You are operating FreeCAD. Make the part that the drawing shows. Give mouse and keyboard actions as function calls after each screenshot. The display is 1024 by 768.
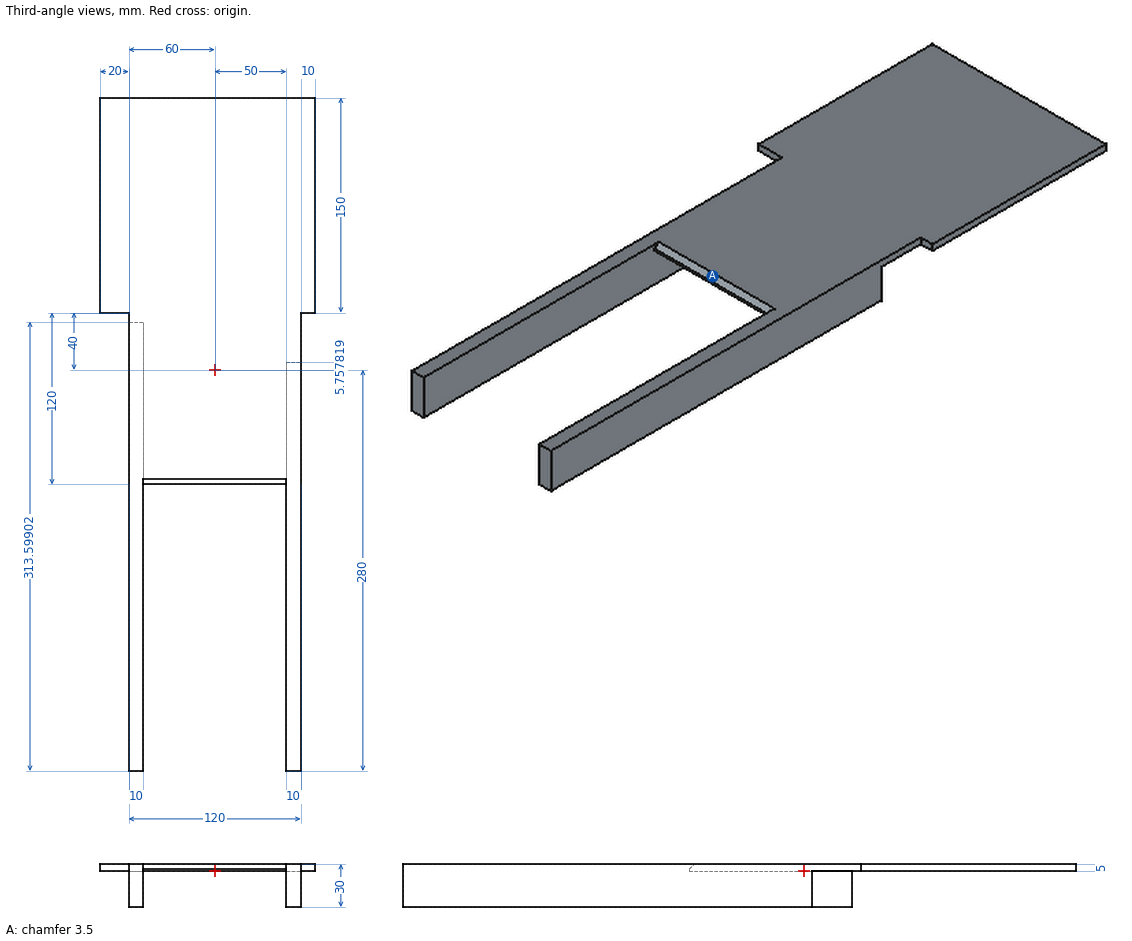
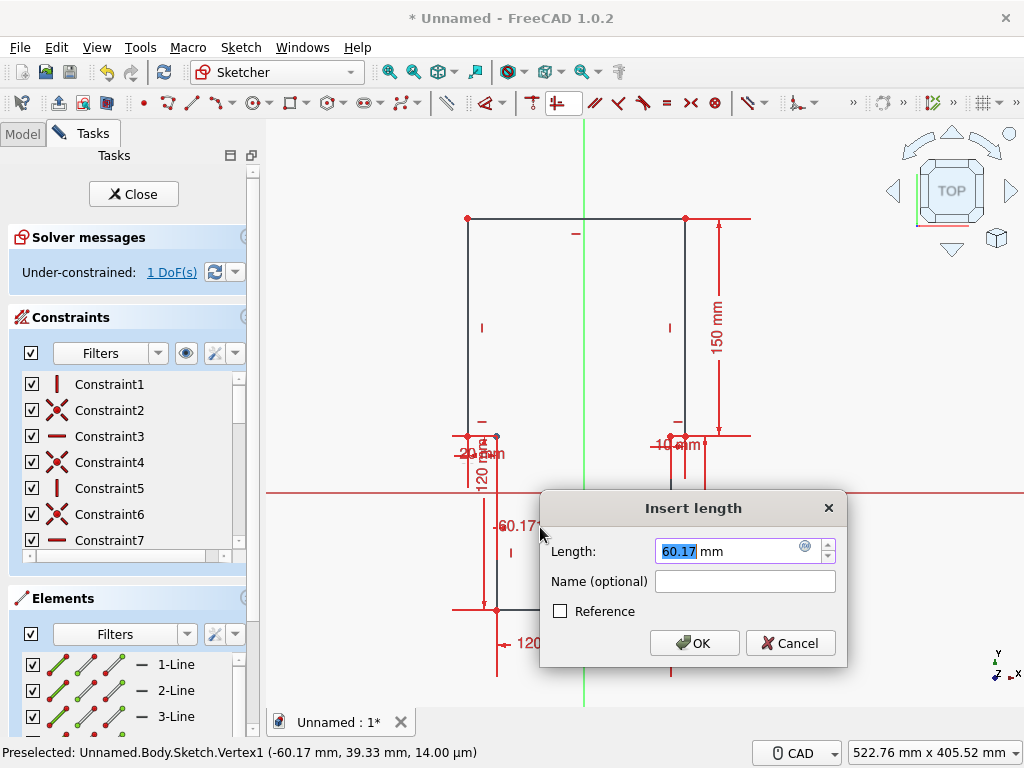
text(60)
key(Return)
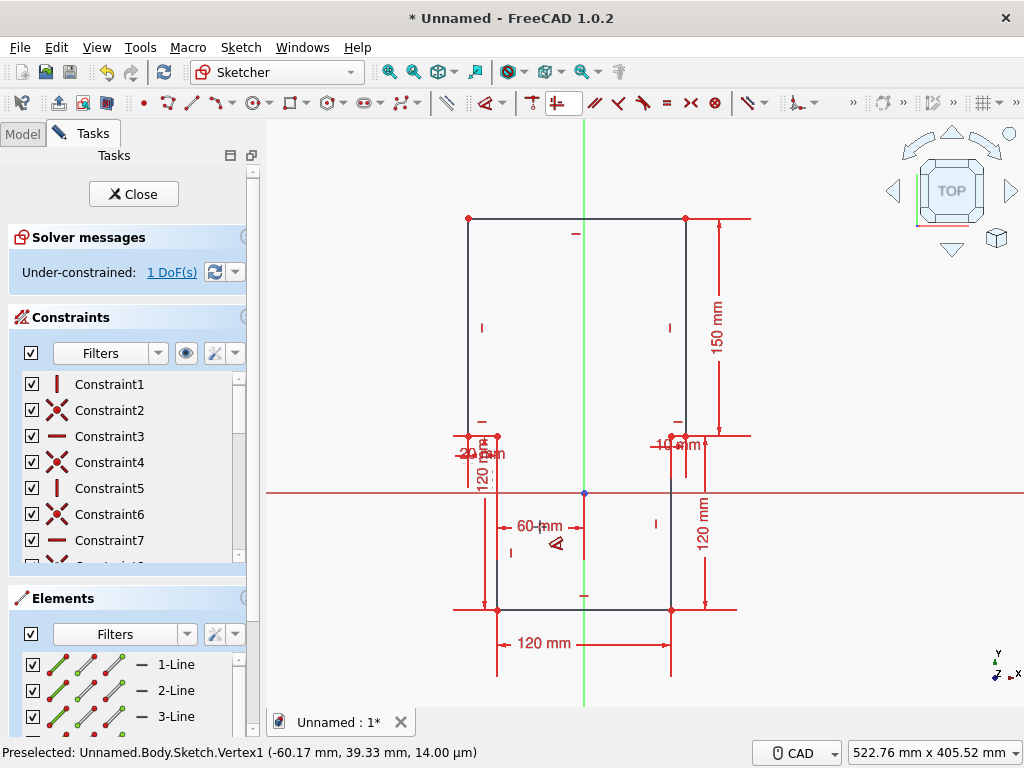
click(497, 436)
click(618, 478)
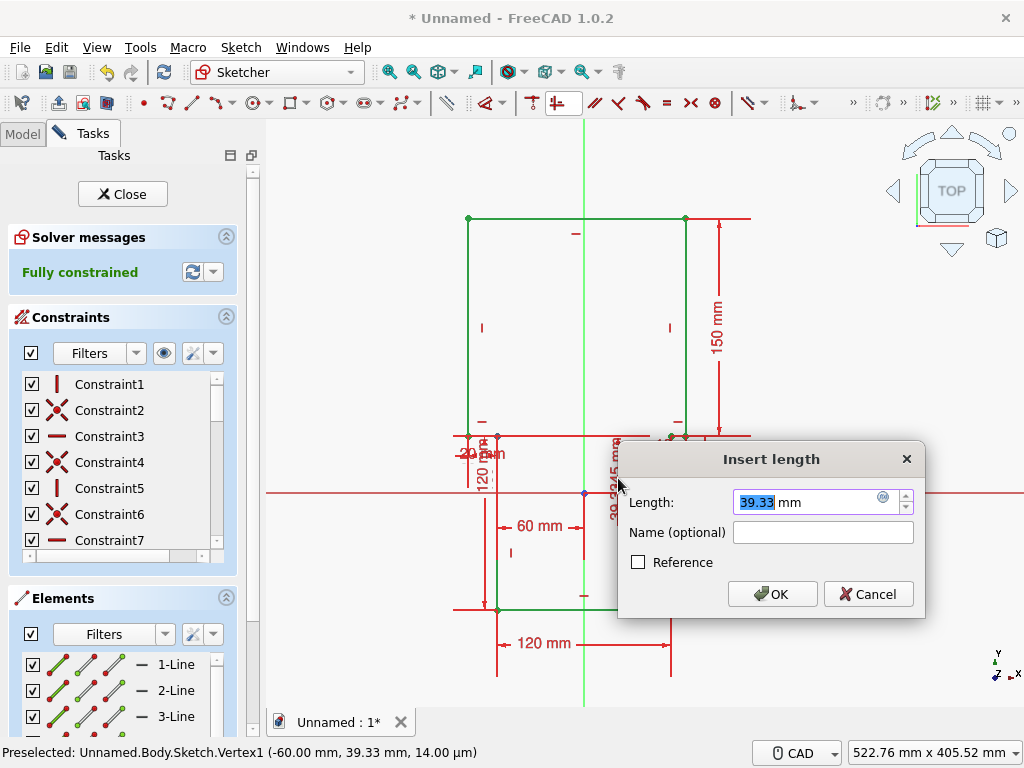
text(40)
key(Return)
key(Escape)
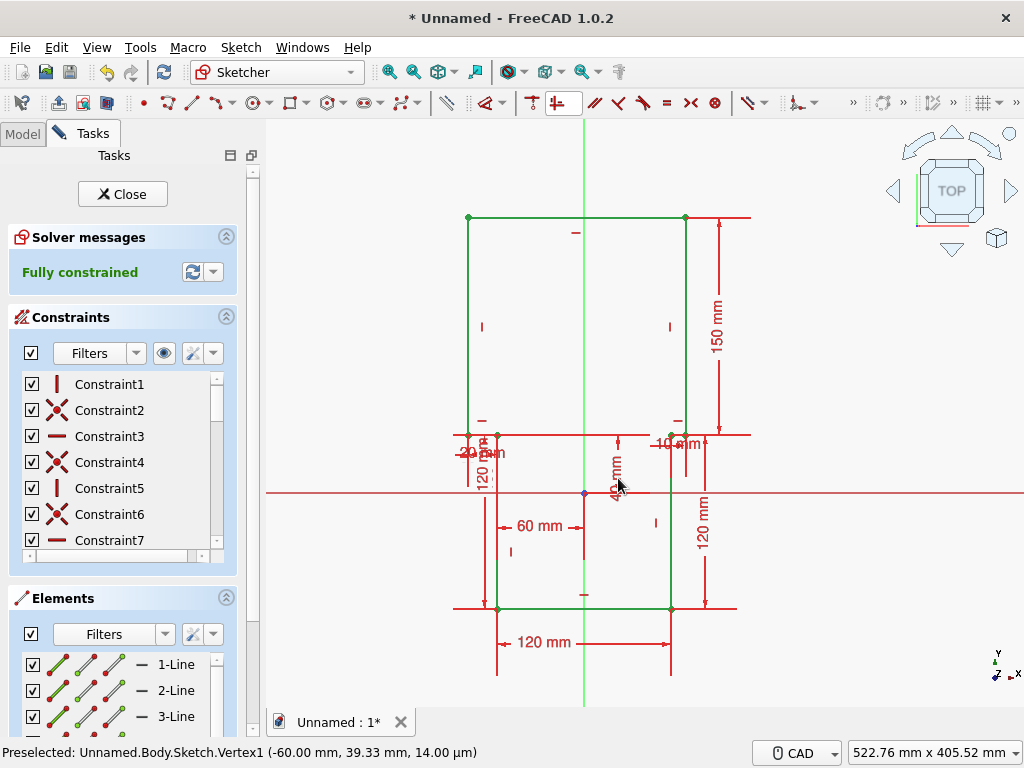
click(123, 194)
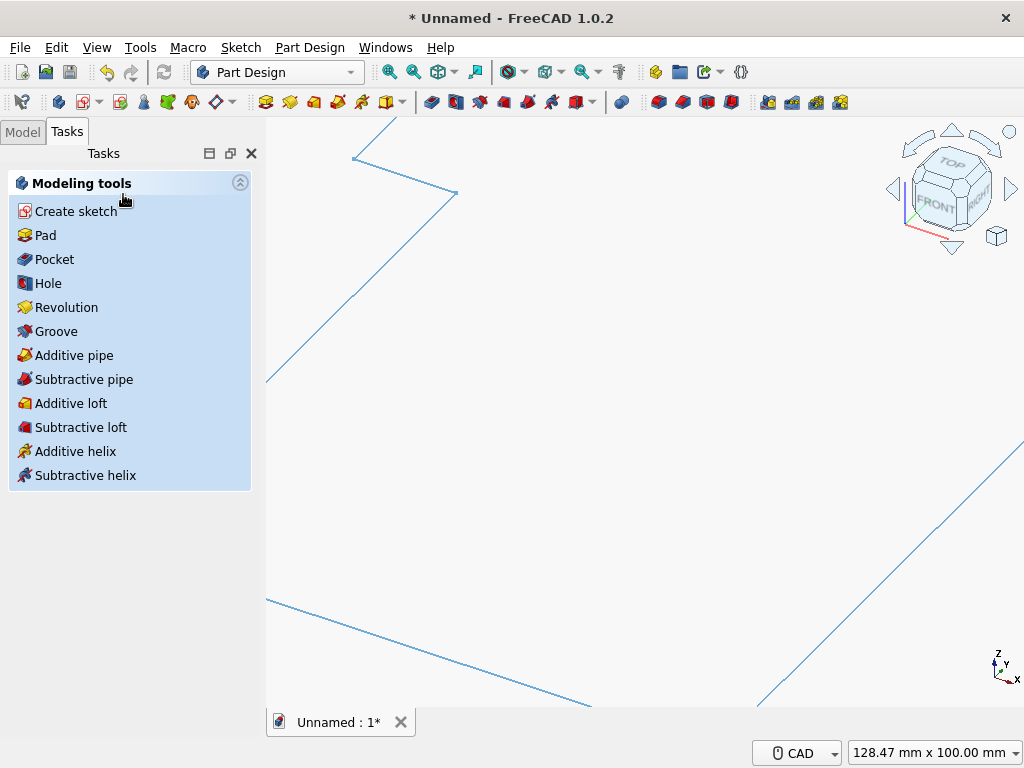
click(266, 102)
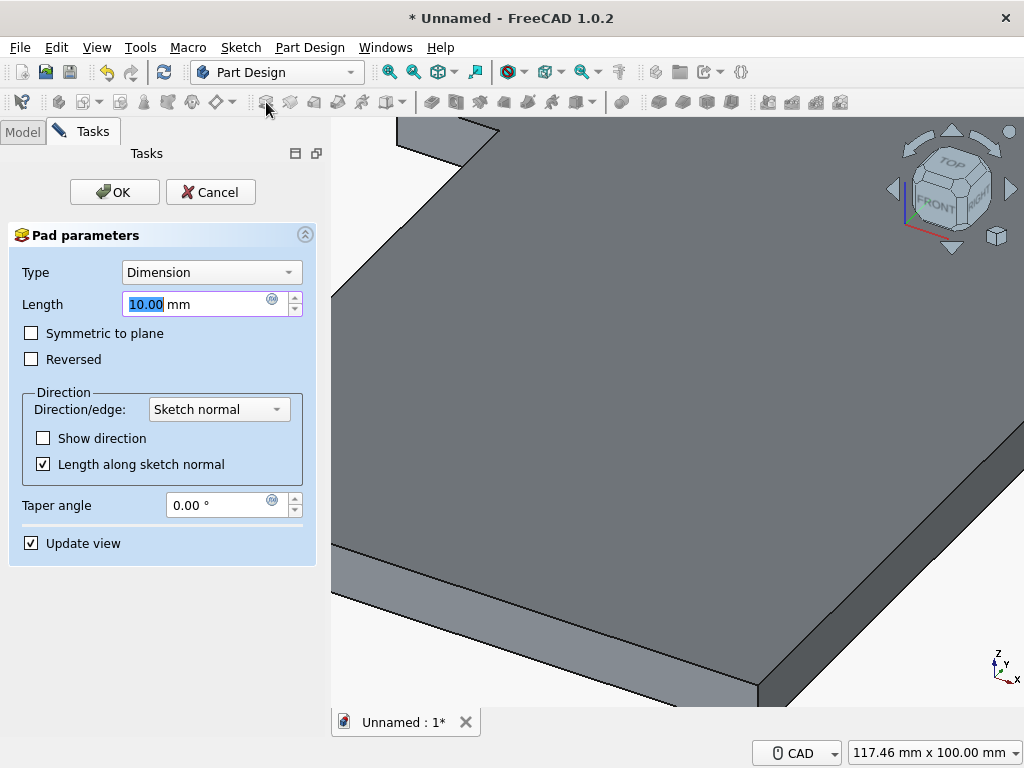
text(5)
key(Tab)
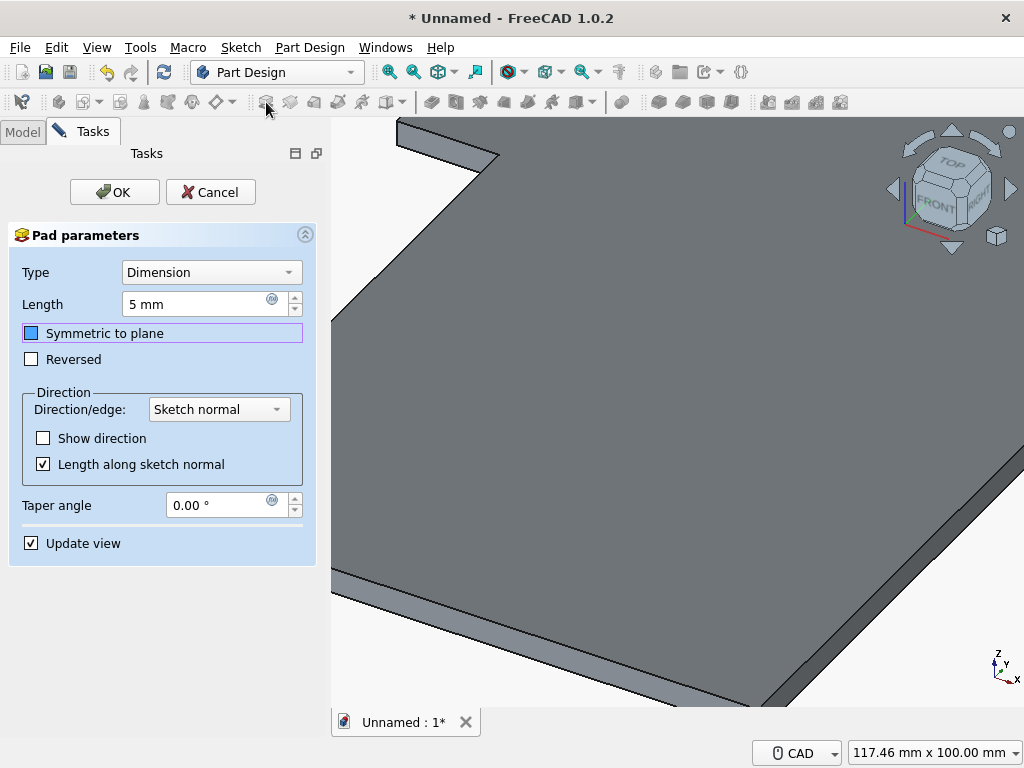
click(115, 192)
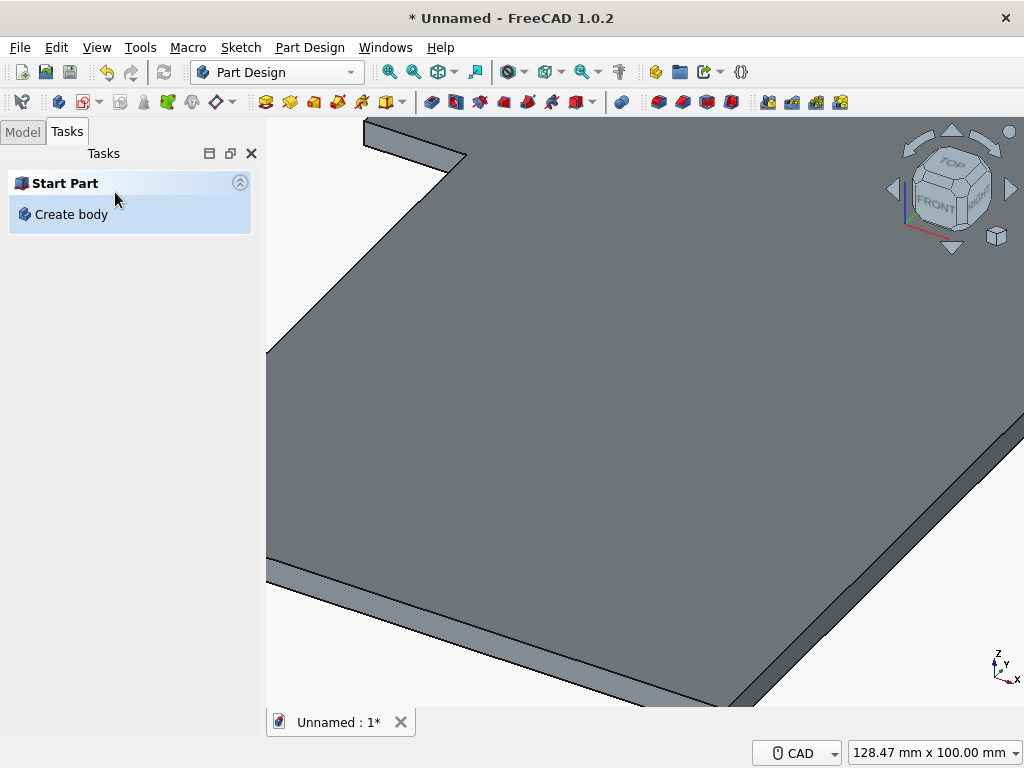
click(390, 72)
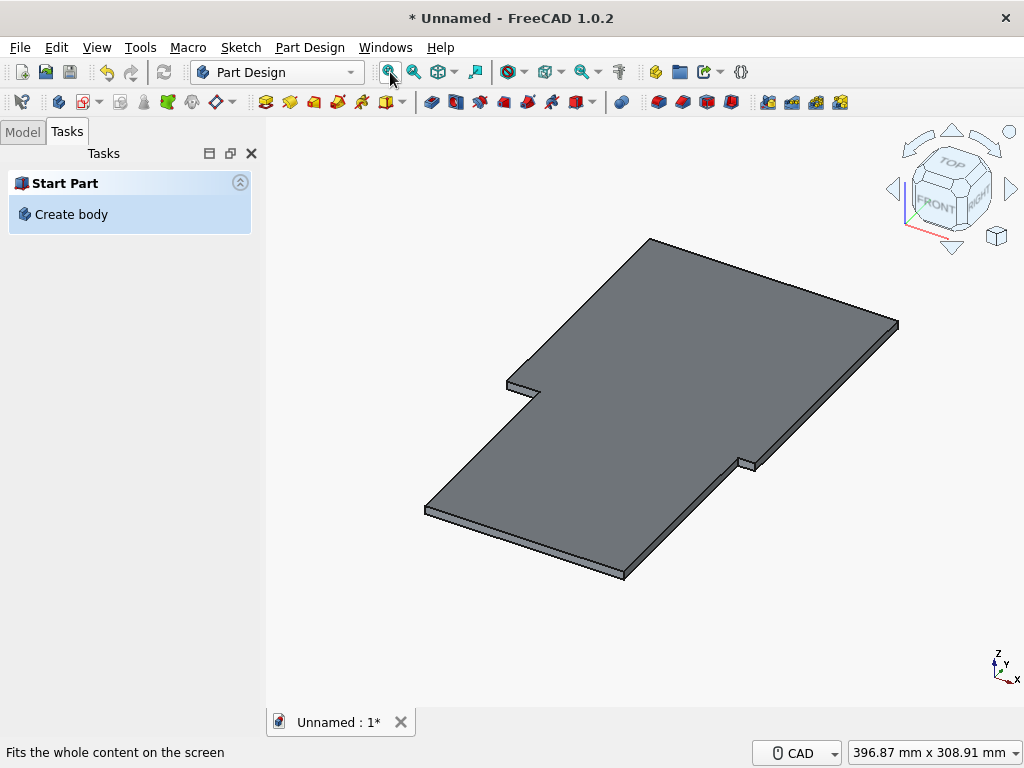
click(682, 370)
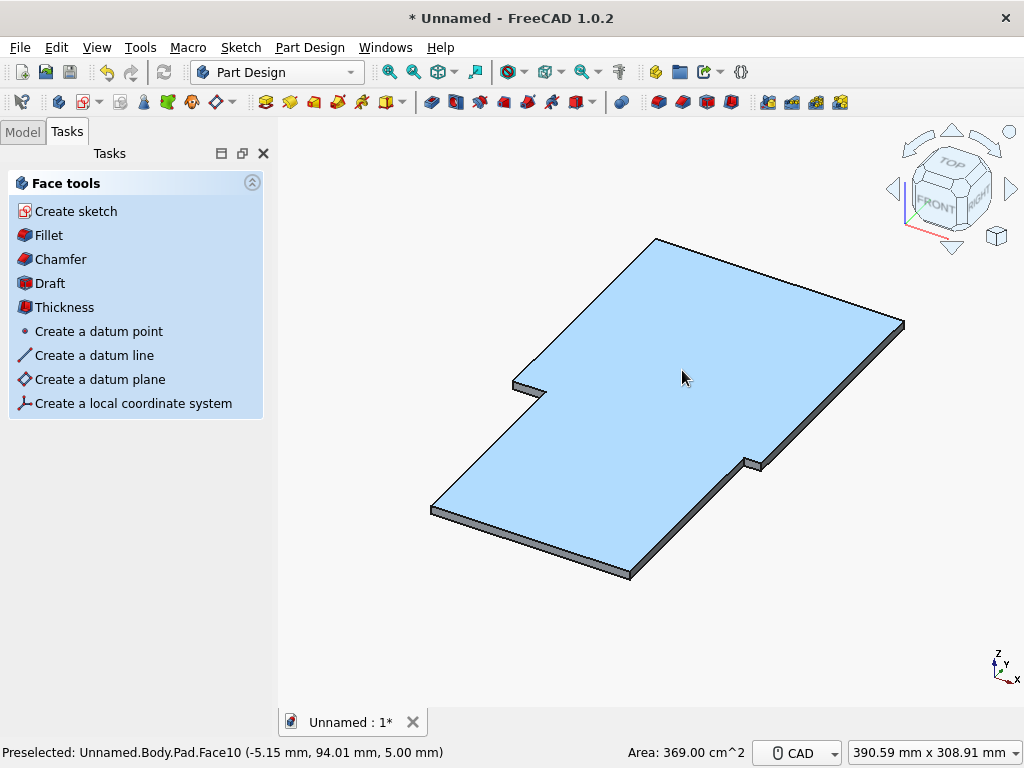
click(84, 102)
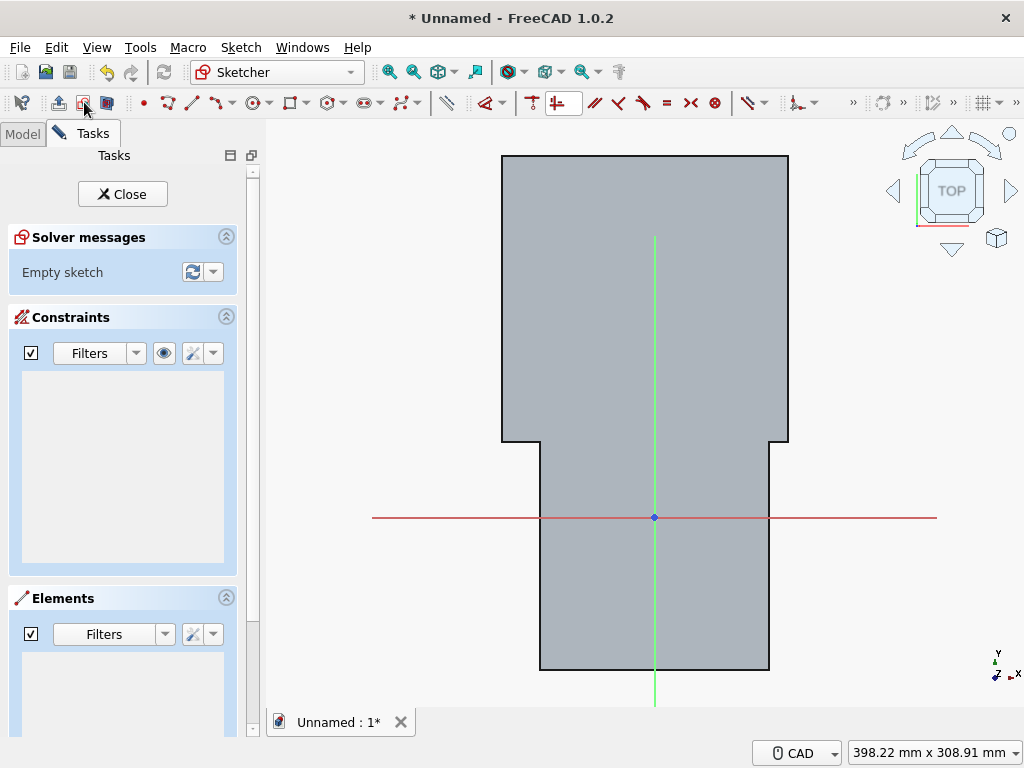
scroll(482, 147, down, 3)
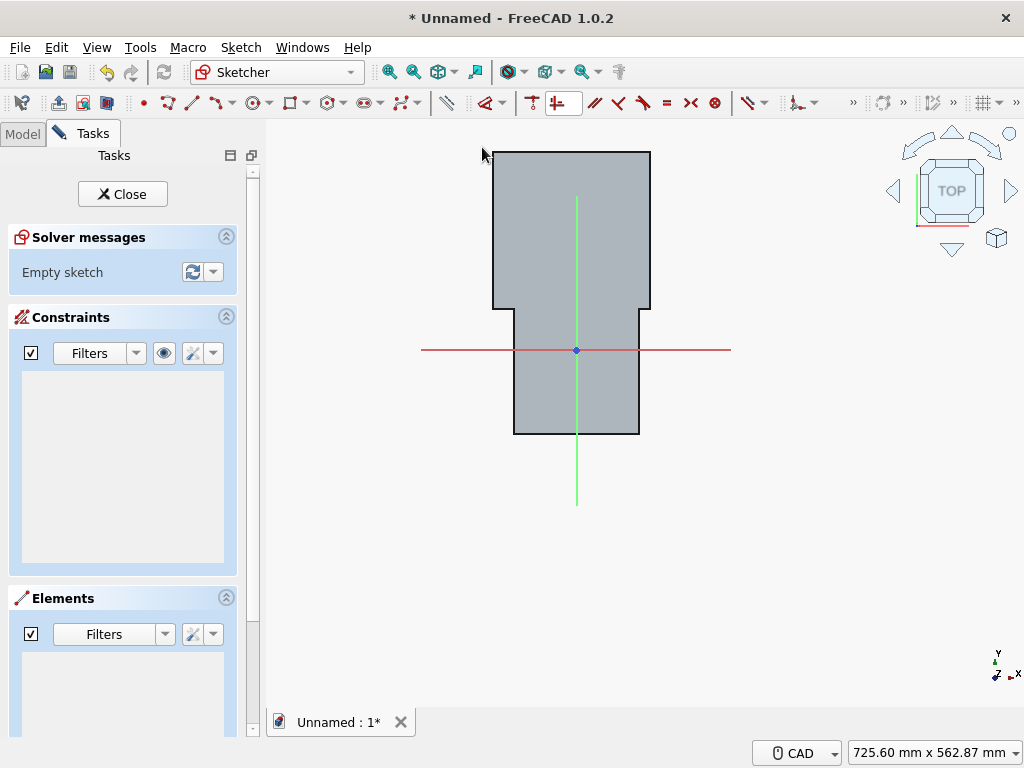
click(290, 104)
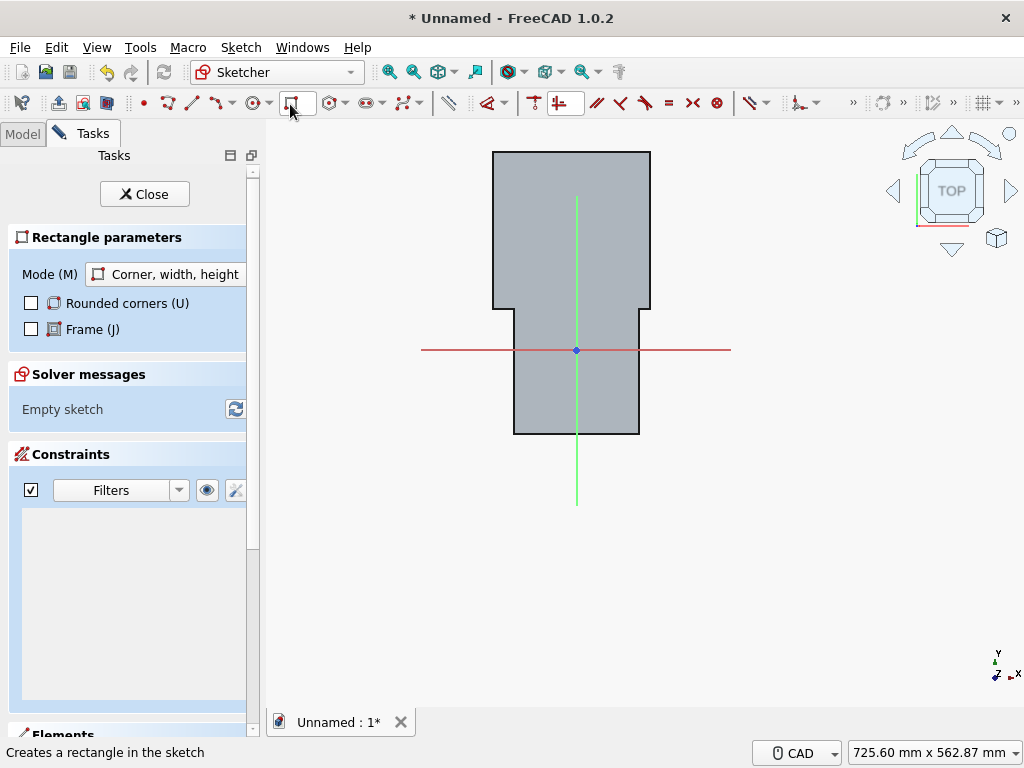
scroll(629, 344, up, 5)